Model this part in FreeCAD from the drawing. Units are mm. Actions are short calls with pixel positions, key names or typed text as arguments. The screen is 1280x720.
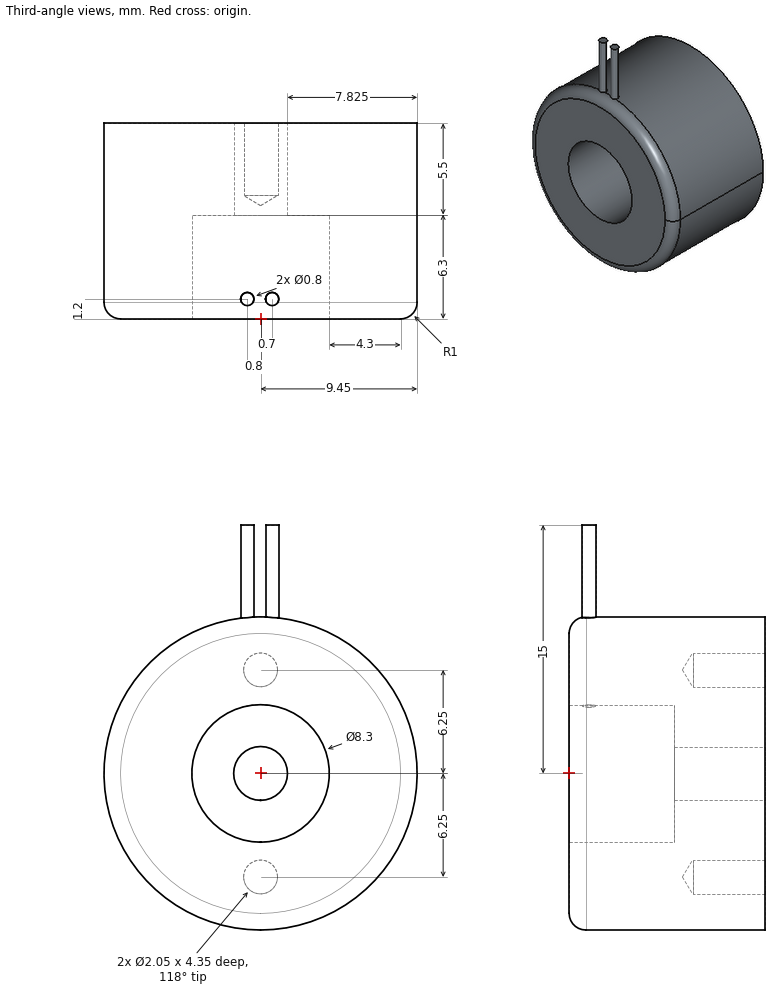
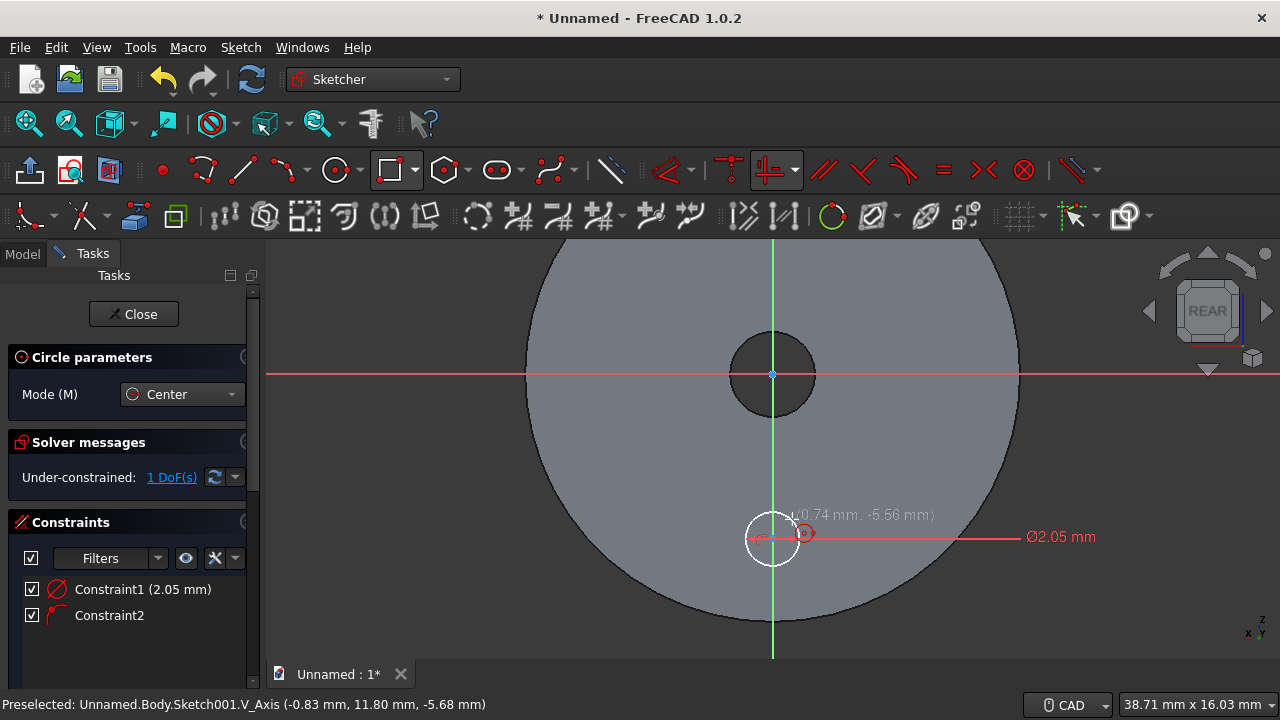
scroll(566, 601, down, 2)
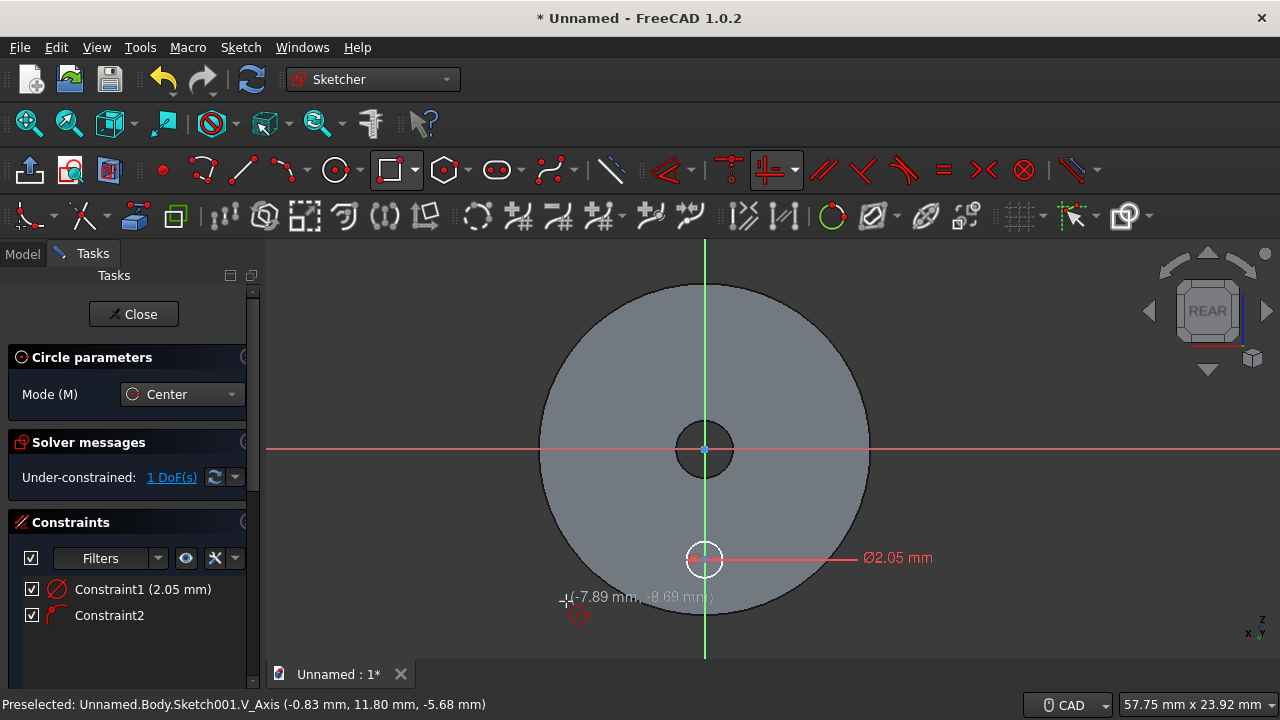
scroll(705, 340, up, 2)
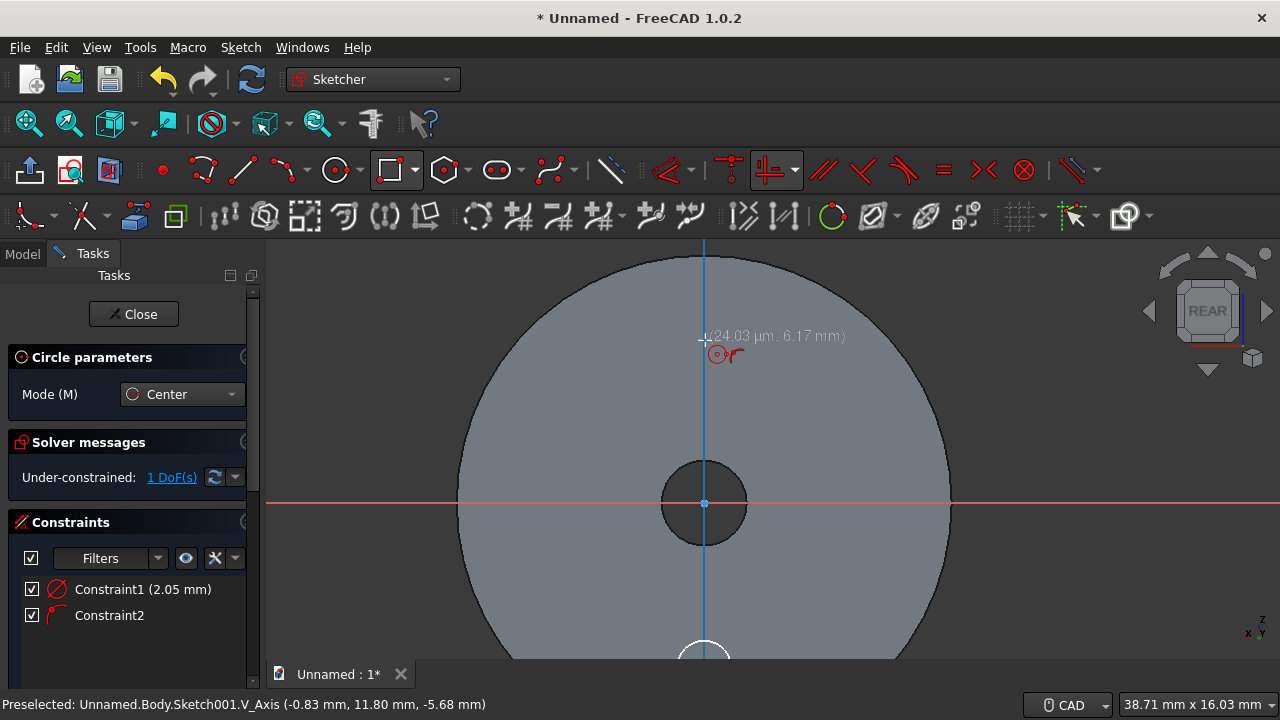
click(704, 339)
move(723, 320)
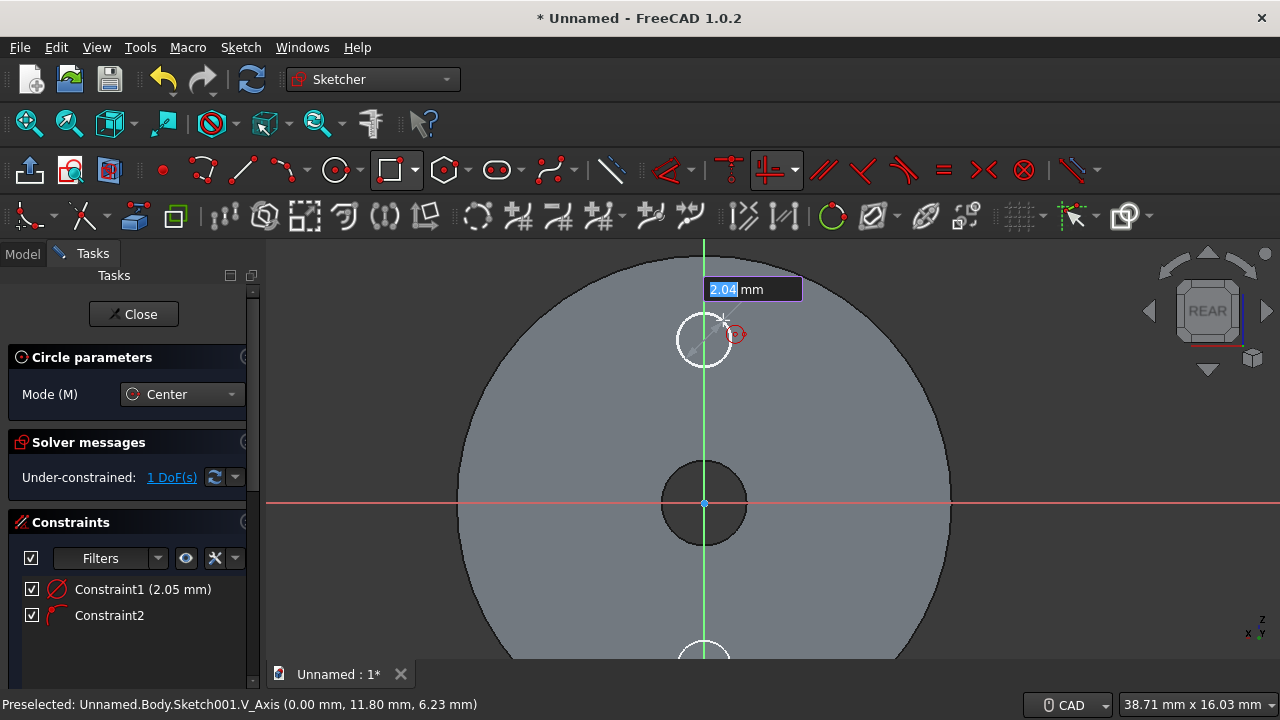
text(2.05)
key(Return)
key(Escape)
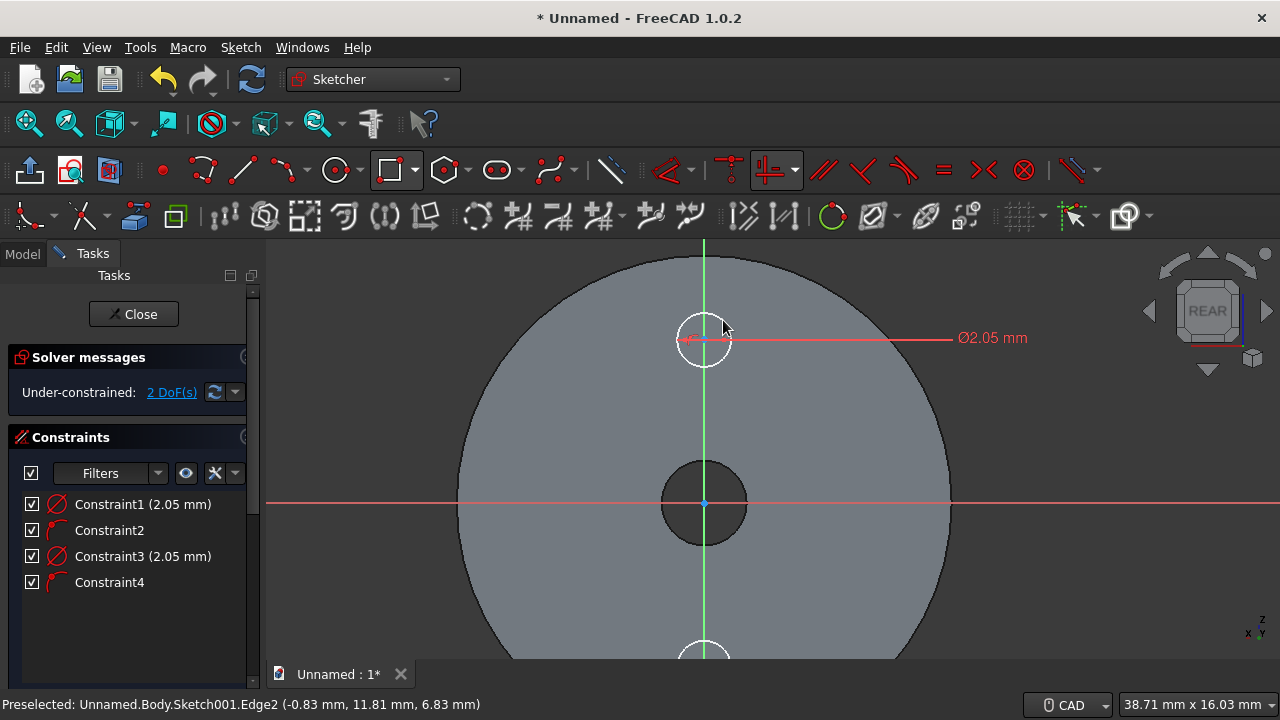
click(666, 170)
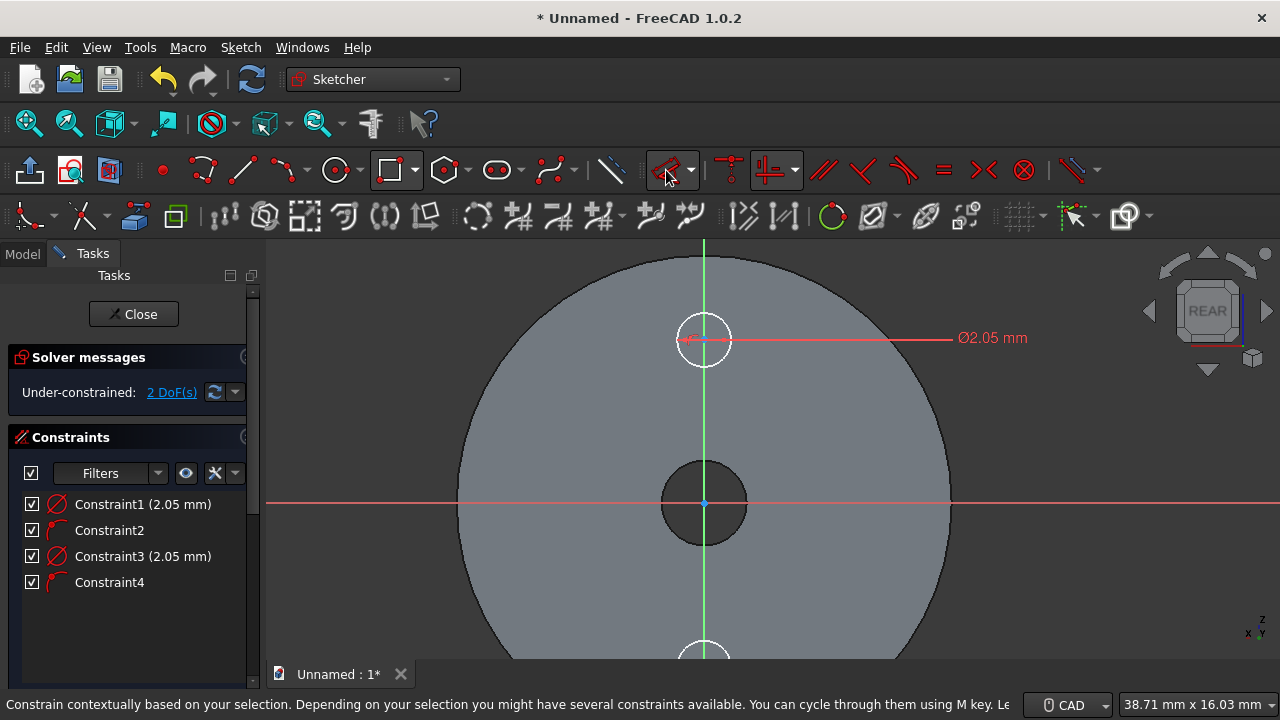
scroll(705, 339, down, 2)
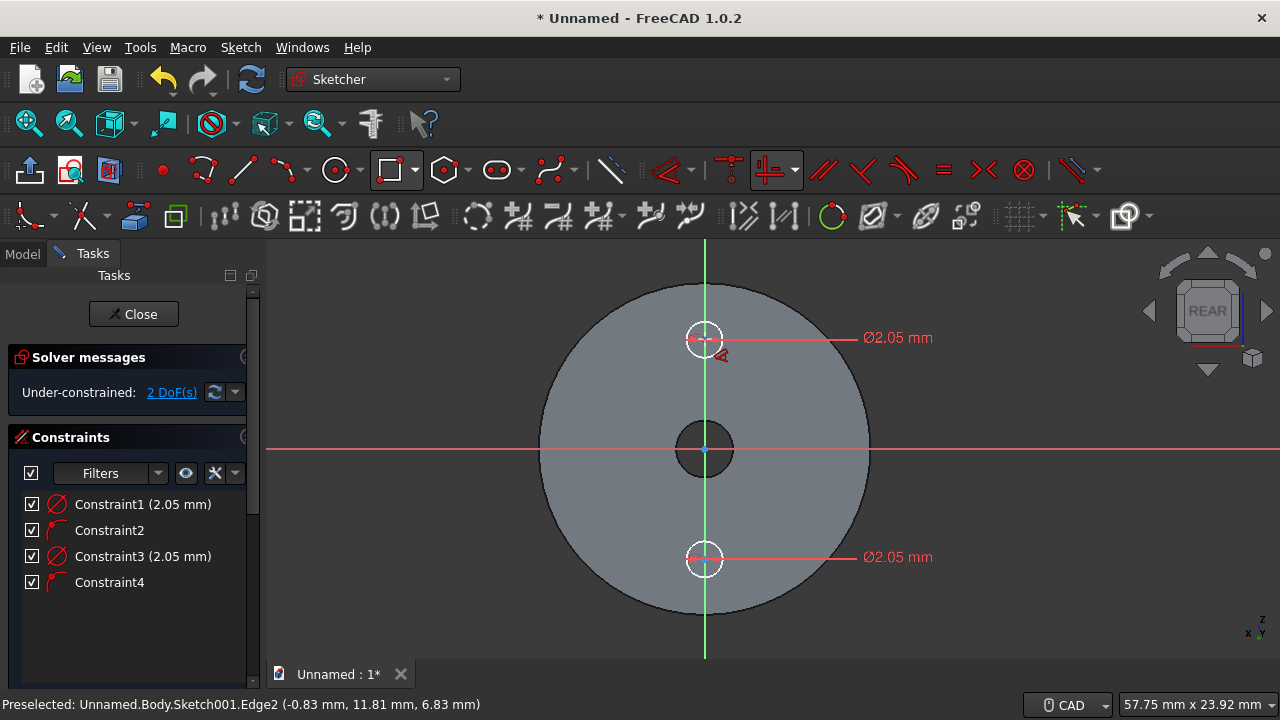
click(705, 559)
click(739, 504)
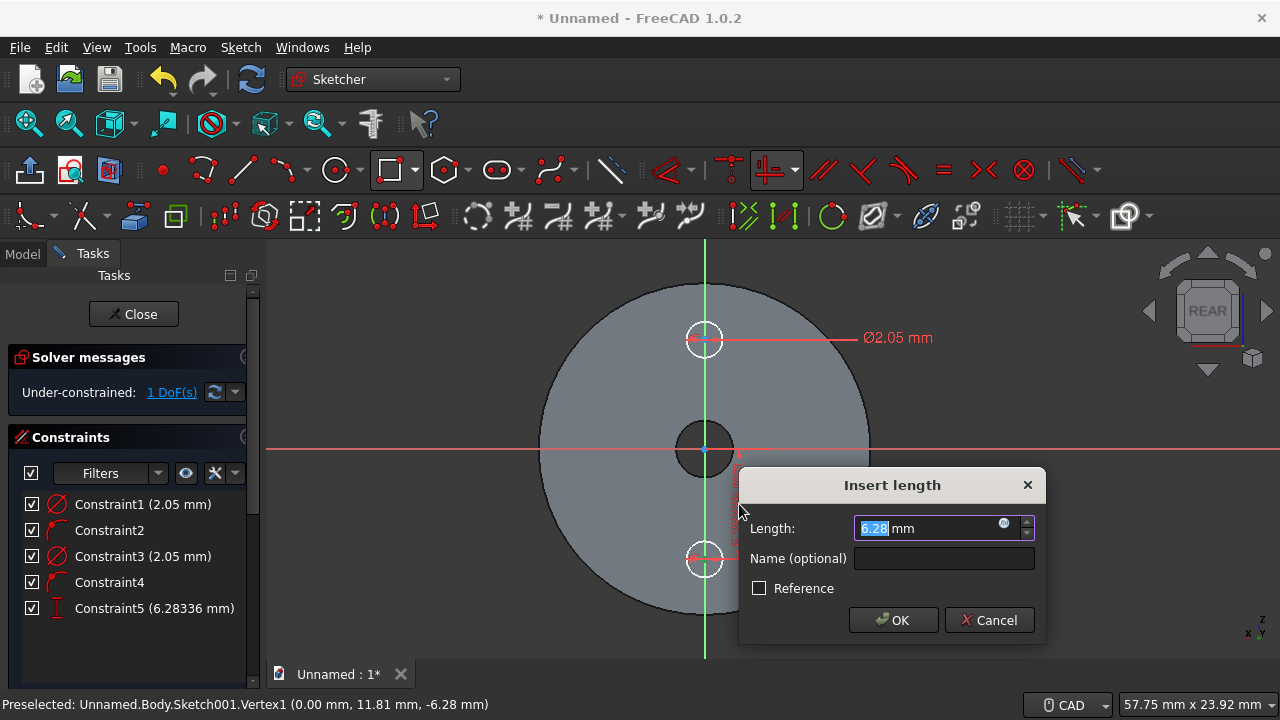
text(6.25)
key(Return)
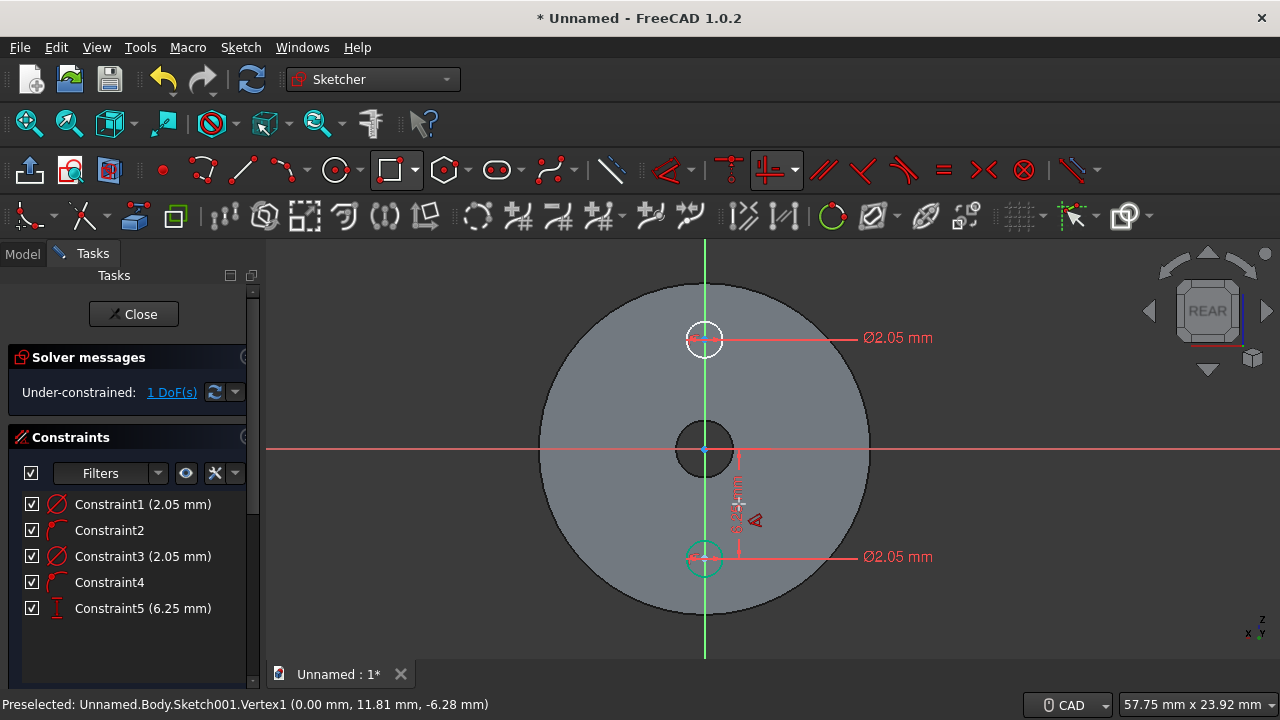
click(705, 340)
click(739, 394)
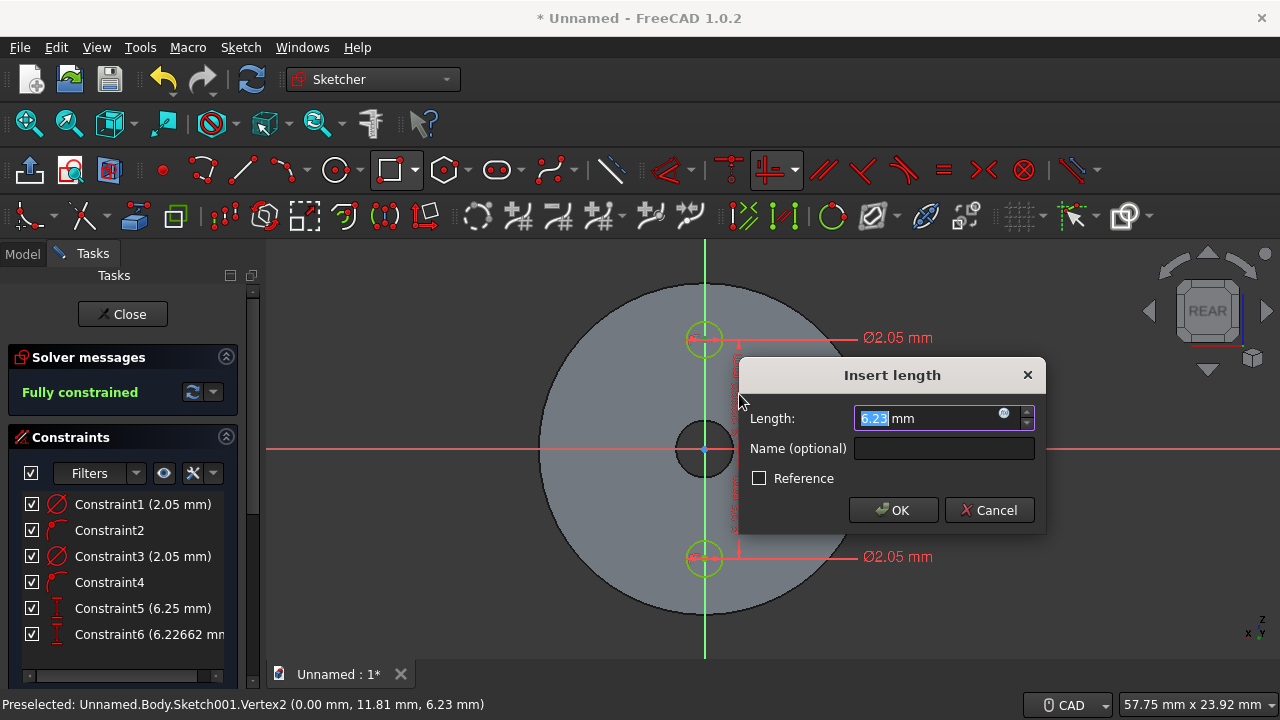
text(6.25)
key(Return)
key(Escape)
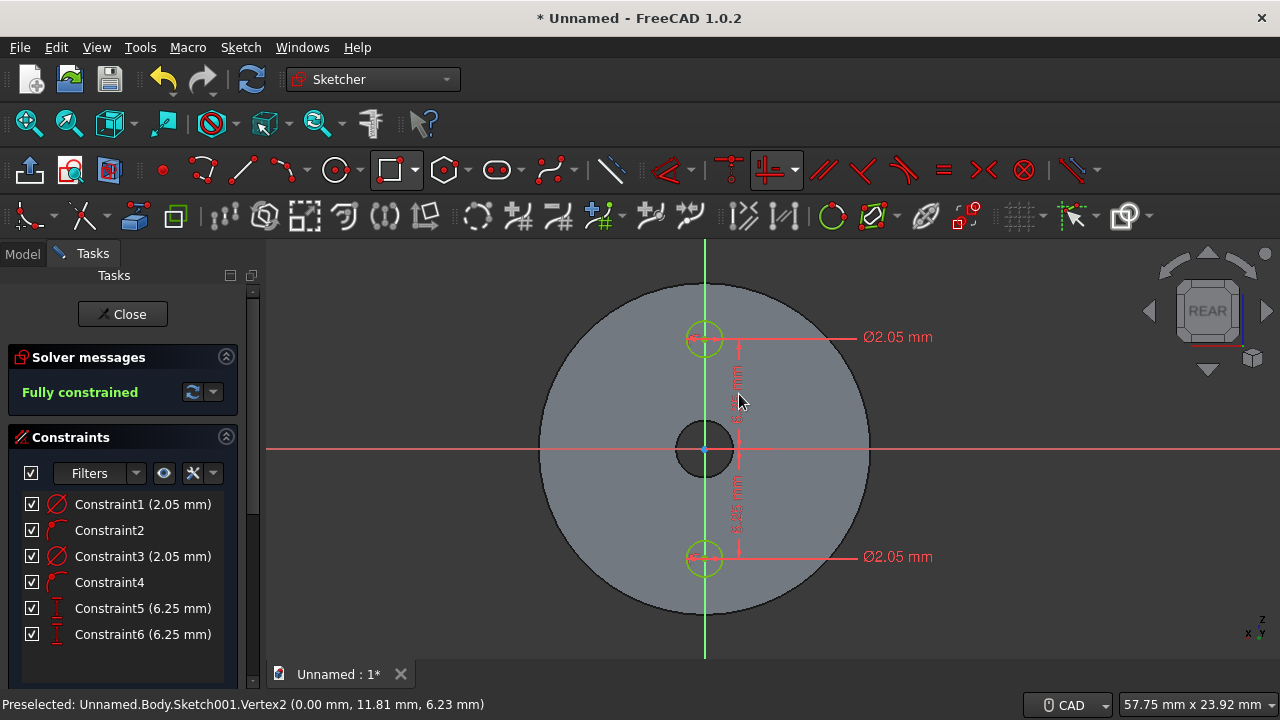
click(123, 314)